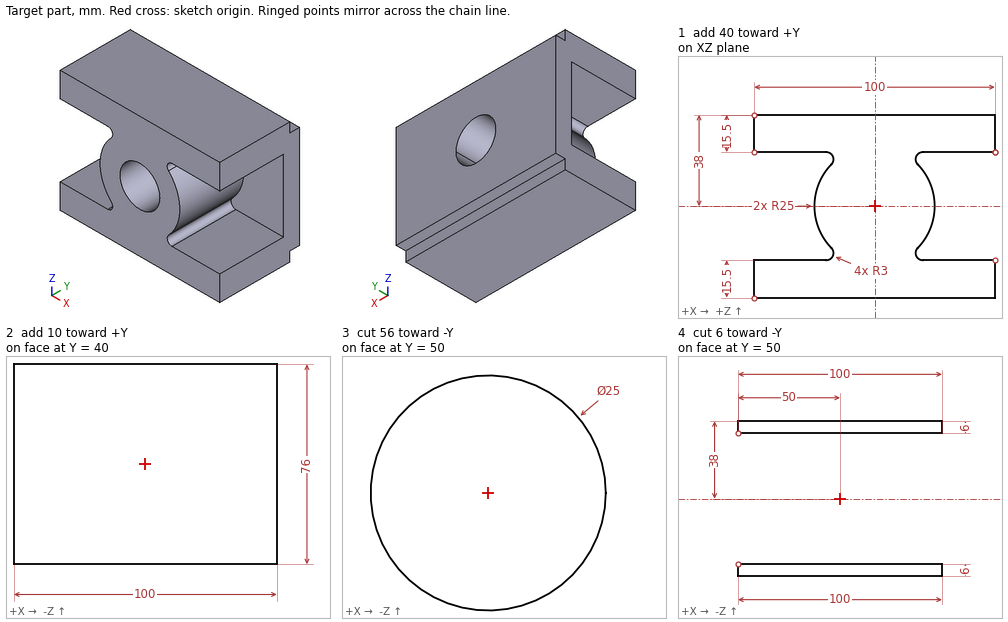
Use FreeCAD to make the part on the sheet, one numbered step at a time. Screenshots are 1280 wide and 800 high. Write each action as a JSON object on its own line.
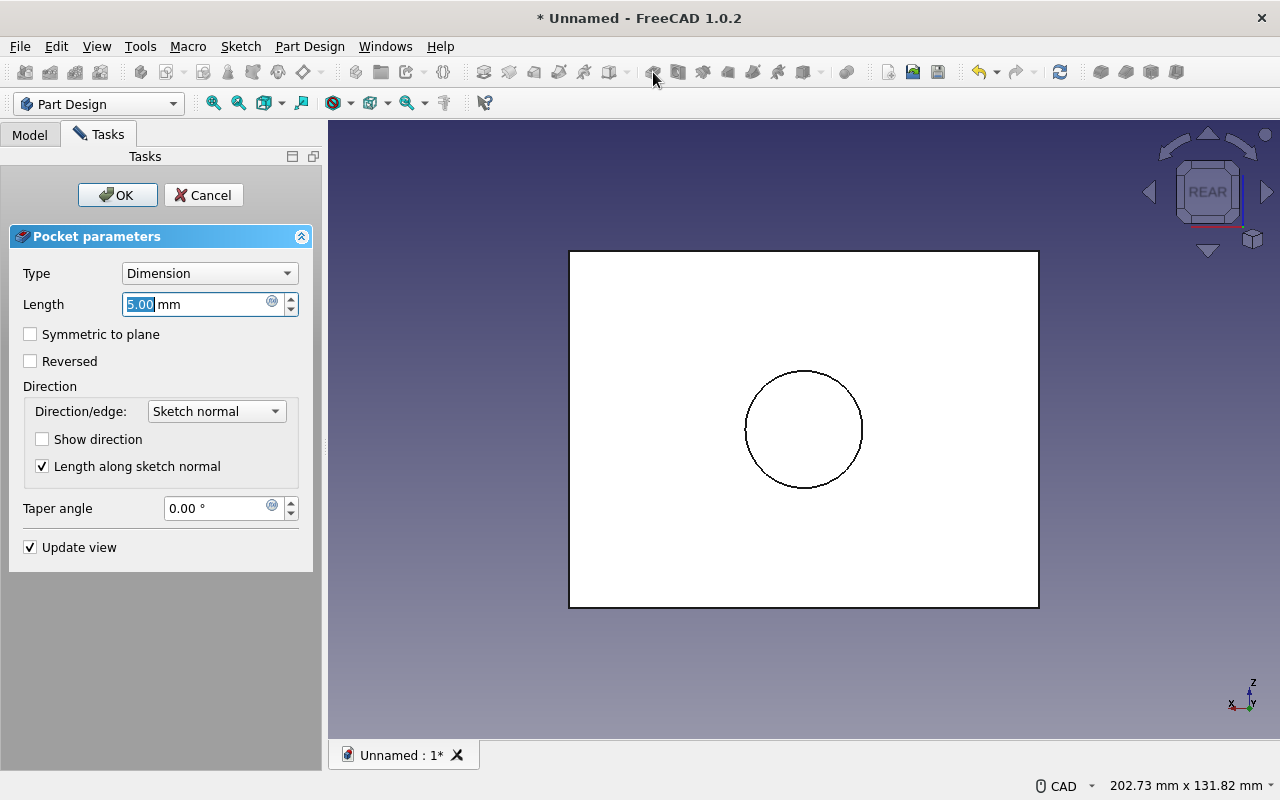
{"action": "type", "text": "56"}
{"action": "key", "text": "Tab"}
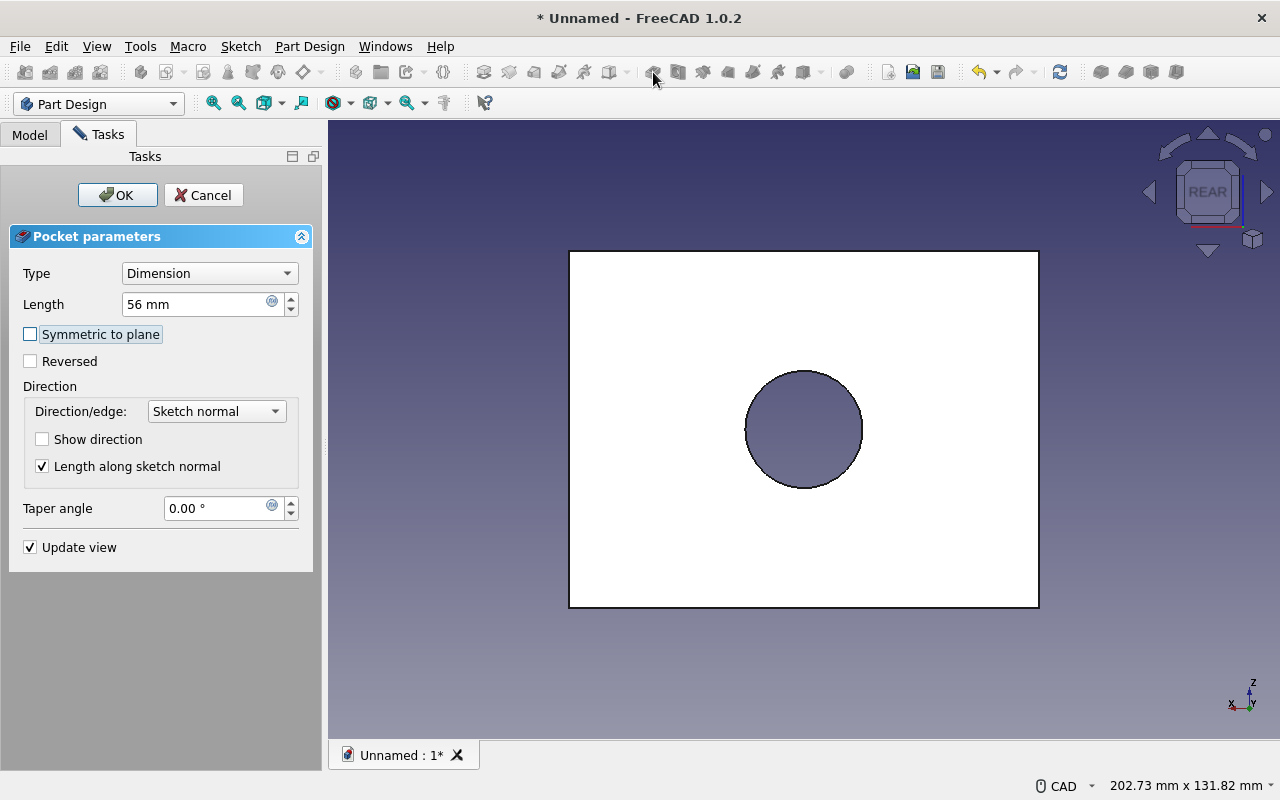
{"action": "left_click", "coordinate": [118, 195]}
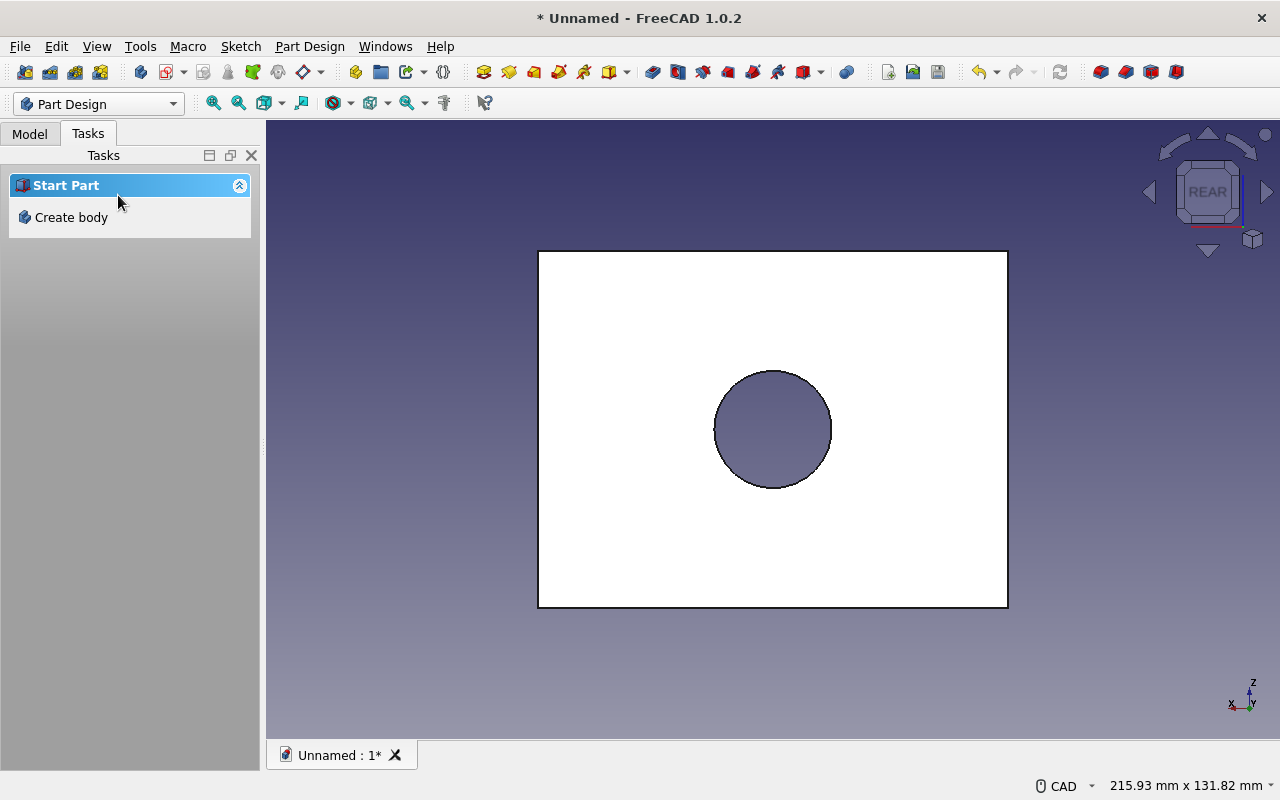
{"action": "left_click", "coordinate": [907, 479]}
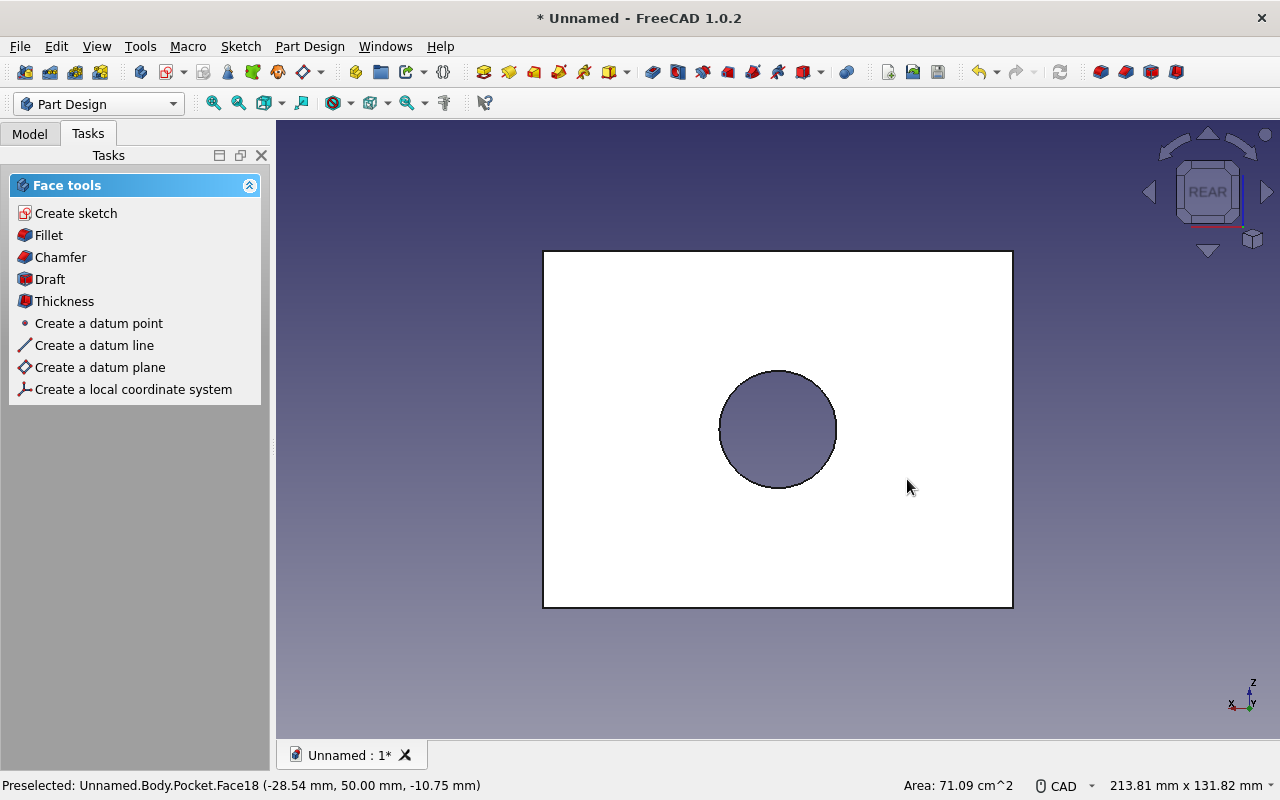
{"action": "left_click", "coordinate": [166, 72]}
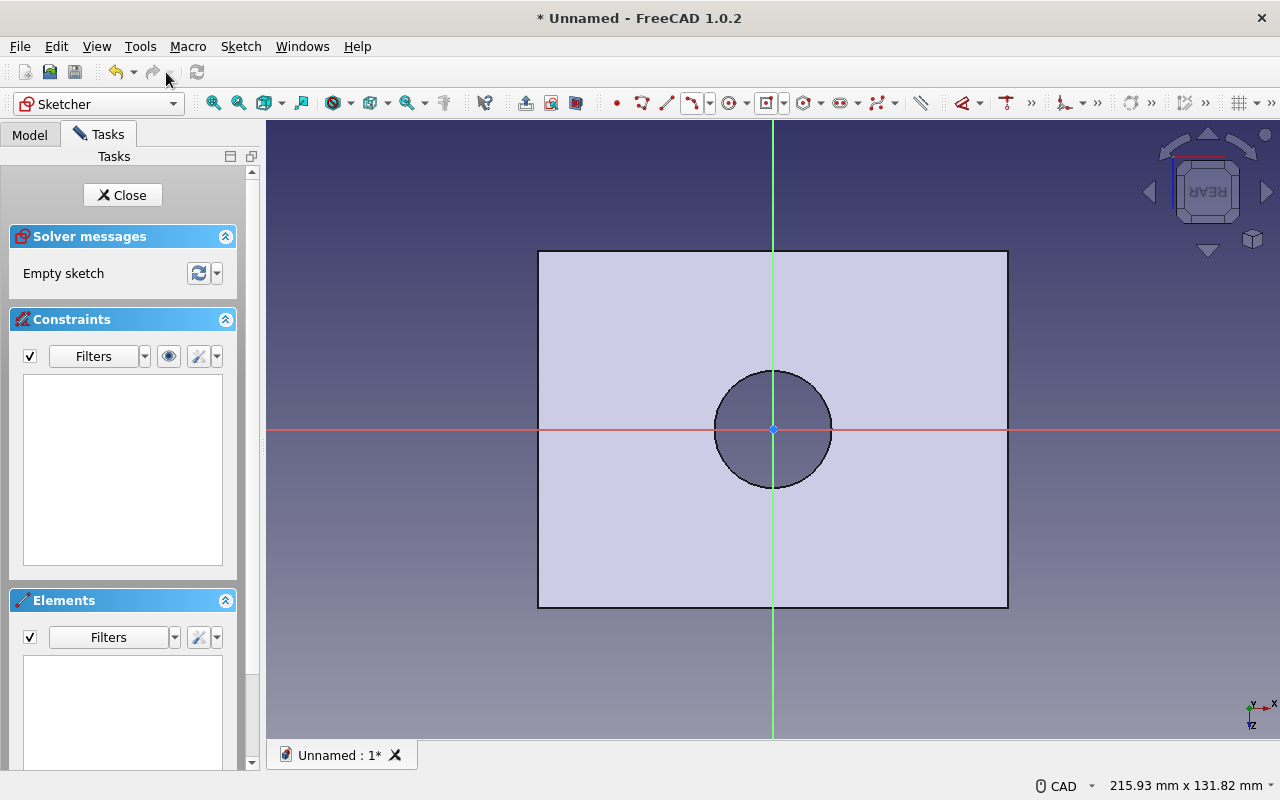
{"action": "left_click", "coordinate": [784, 104]}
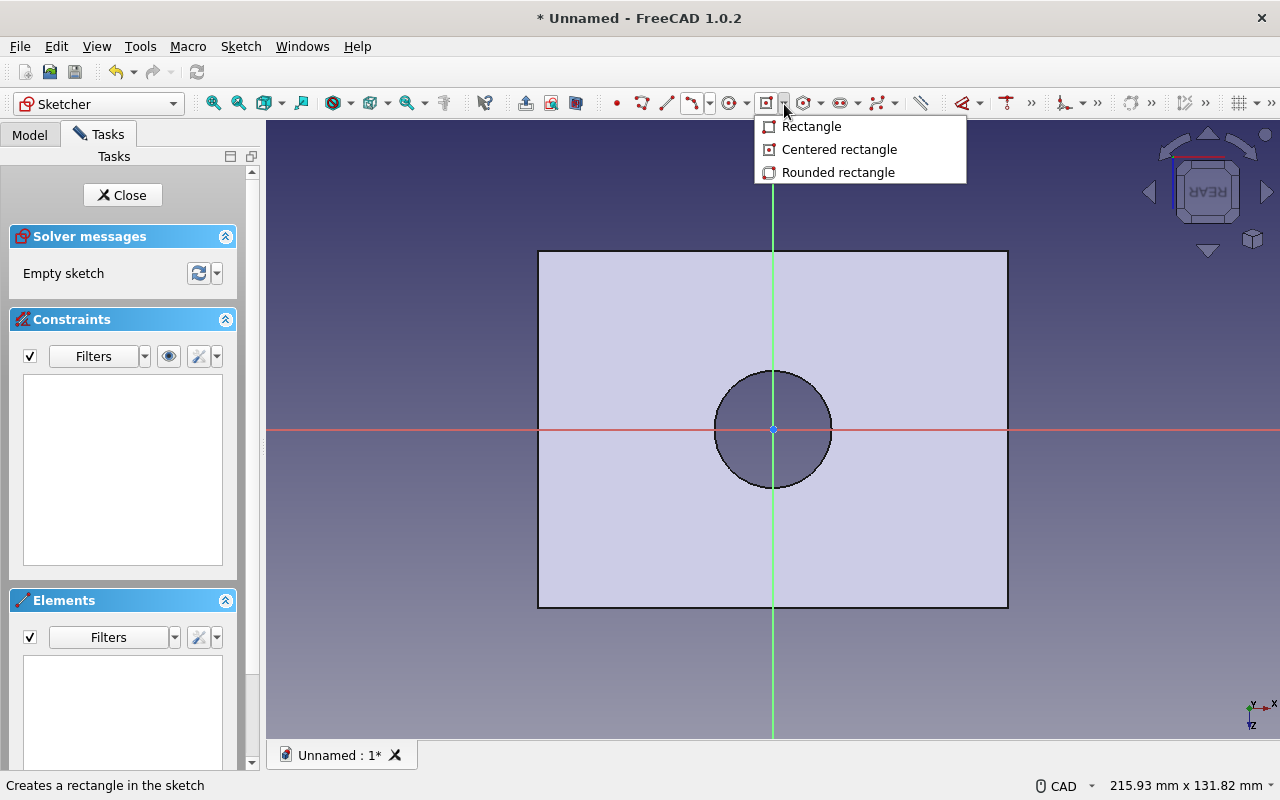
{"action": "left_click", "coordinate": [860, 126]}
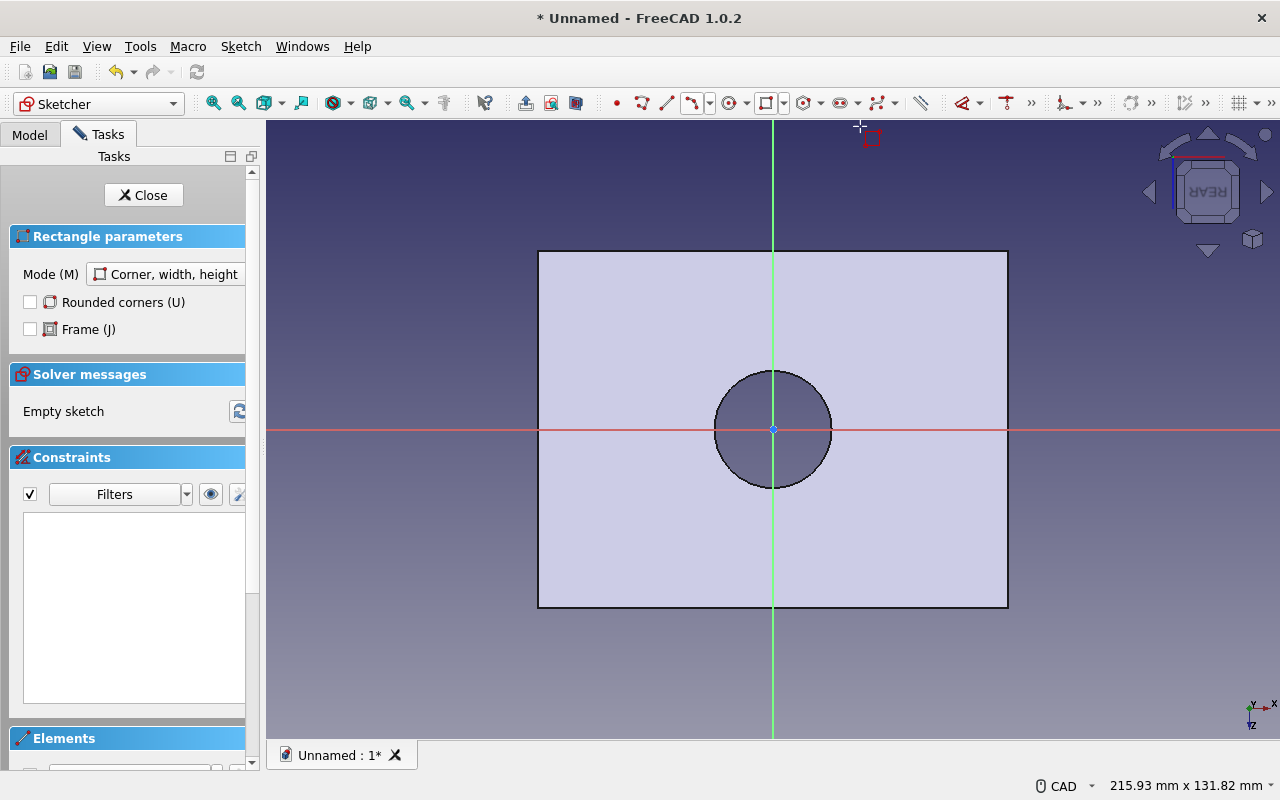
{"action": "left_click", "coordinate": [538, 251]}
{"action": "mouse_move", "coordinate": [1008, 279]}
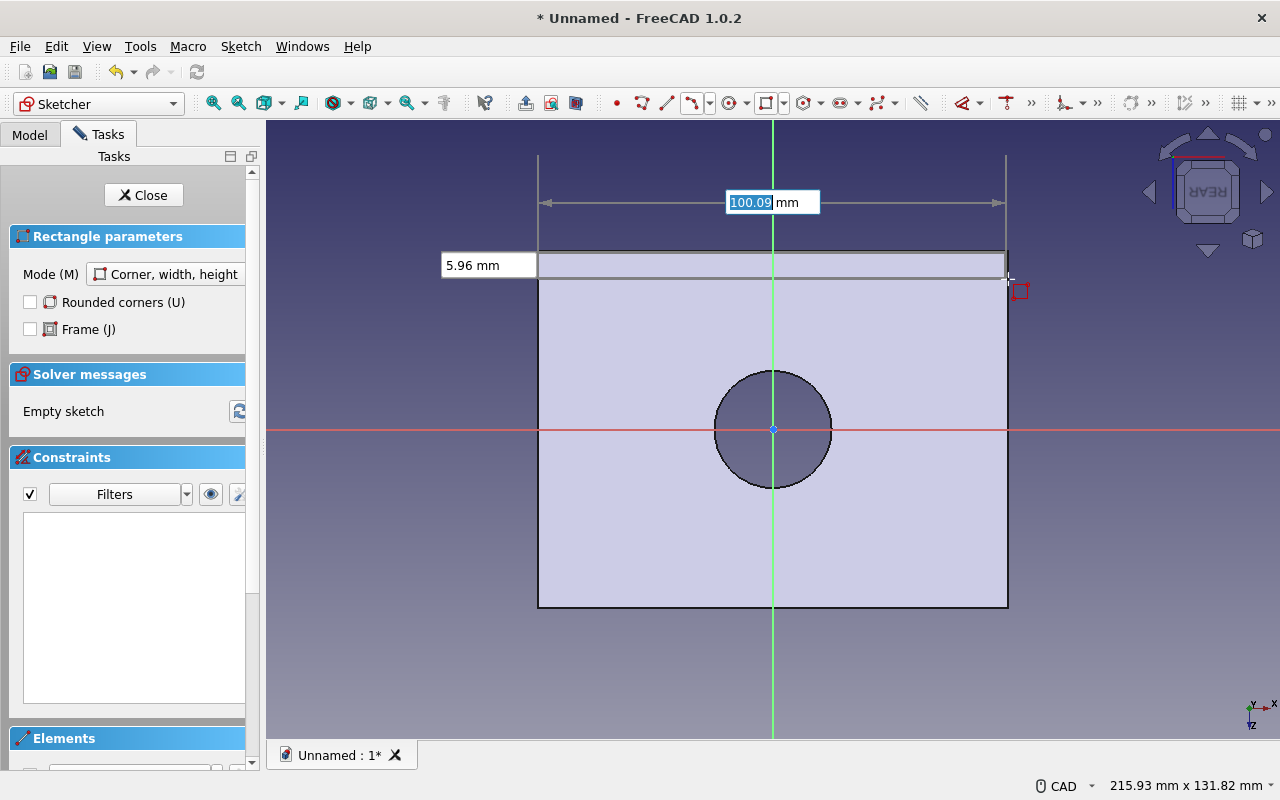
{"action": "type", "text": "100"}
{"action": "key", "text": "Tab"}
{"action": "type", "text": "6"}
{"action": "key", "text": "Return"}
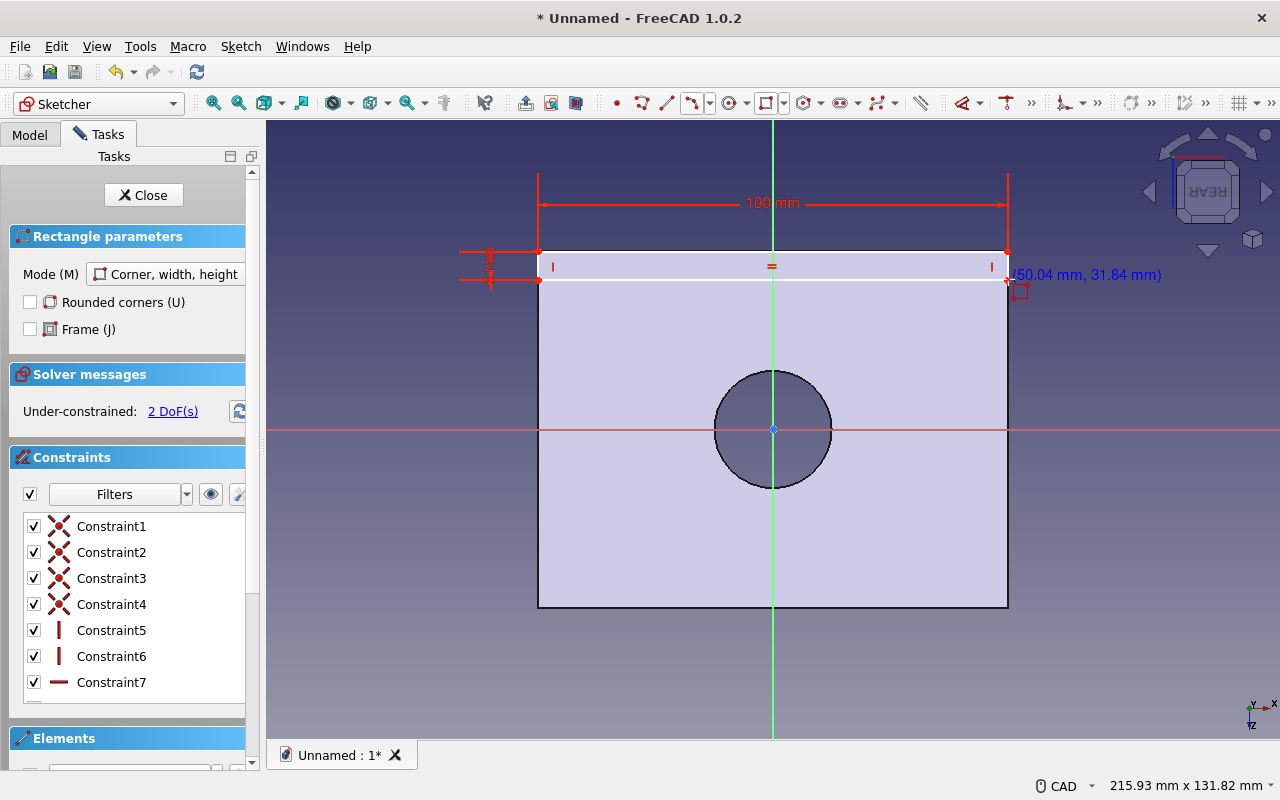
{"action": "left_click", "coordinate": [538, 580]}
{"action": "mouse_move", "coordinate": [1008, 608]}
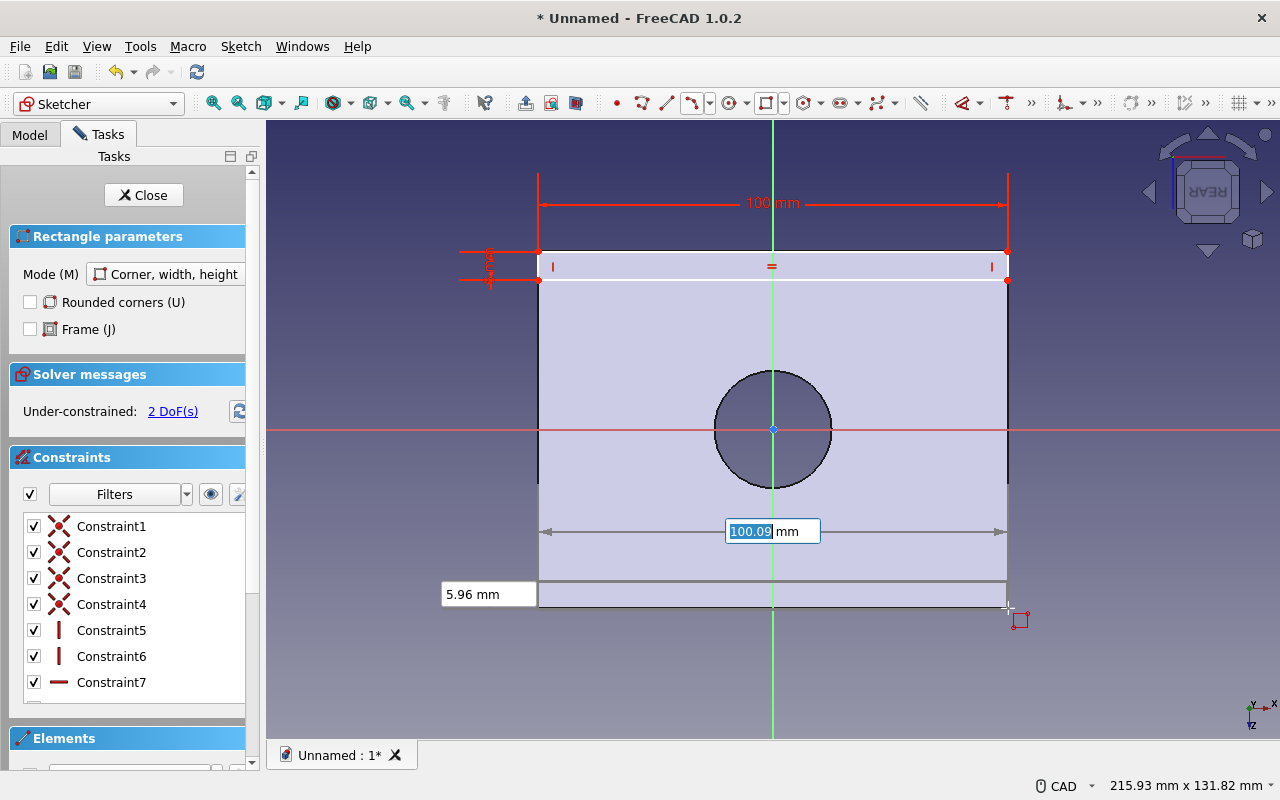
{"action": "type", "text": "100"}
{"action": "key", "text": "Tab"}
{"action": "type", "text": "6"}
{"action": "key", "text": "Return"}
{"action": "key", "text": "Escape"}